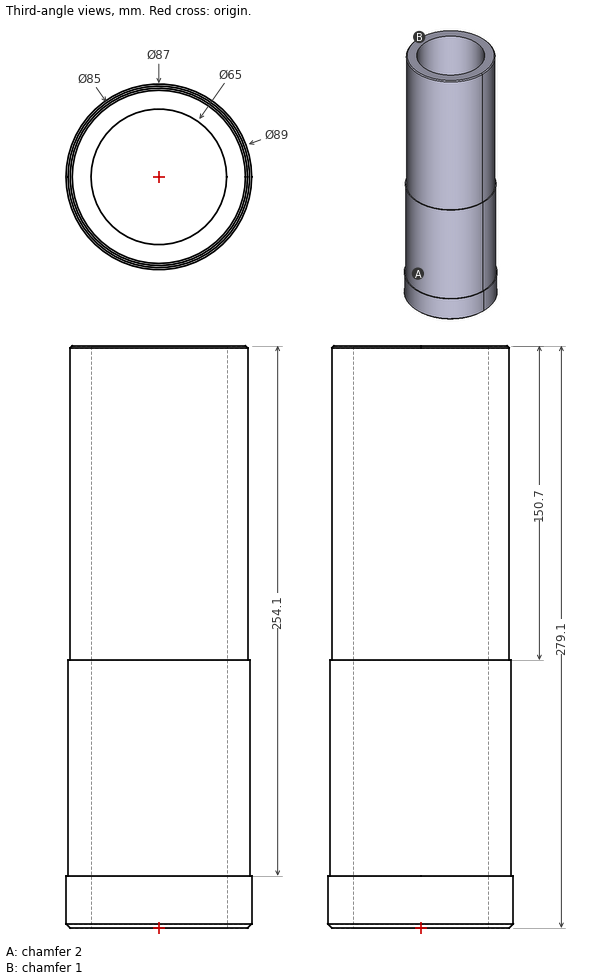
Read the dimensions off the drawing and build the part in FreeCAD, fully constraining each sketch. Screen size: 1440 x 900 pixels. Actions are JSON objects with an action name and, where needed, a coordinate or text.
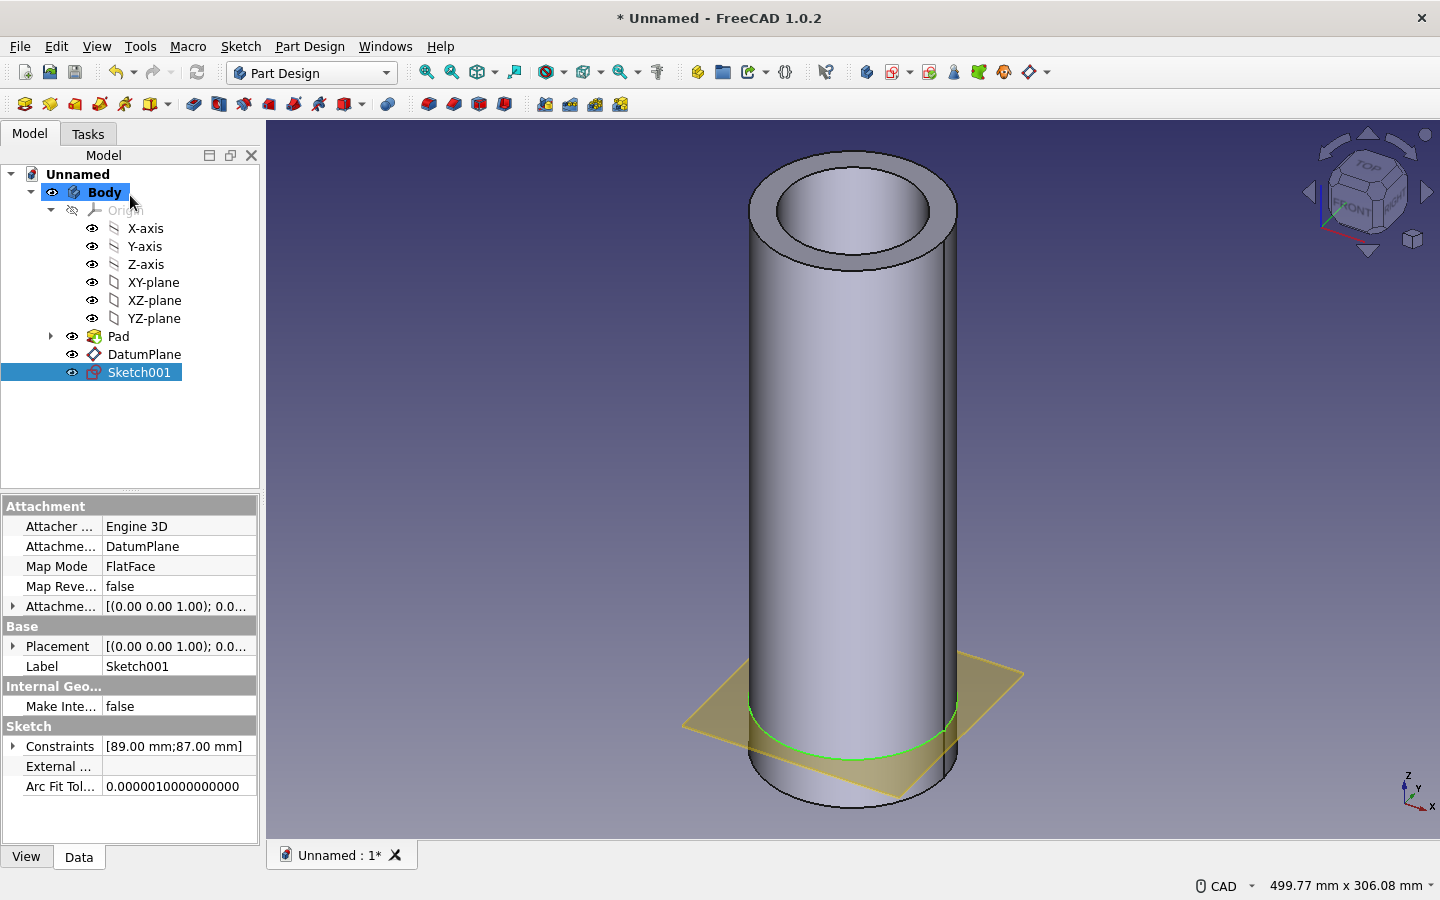
{"action": "left_click", "coordinate": [194, 104]}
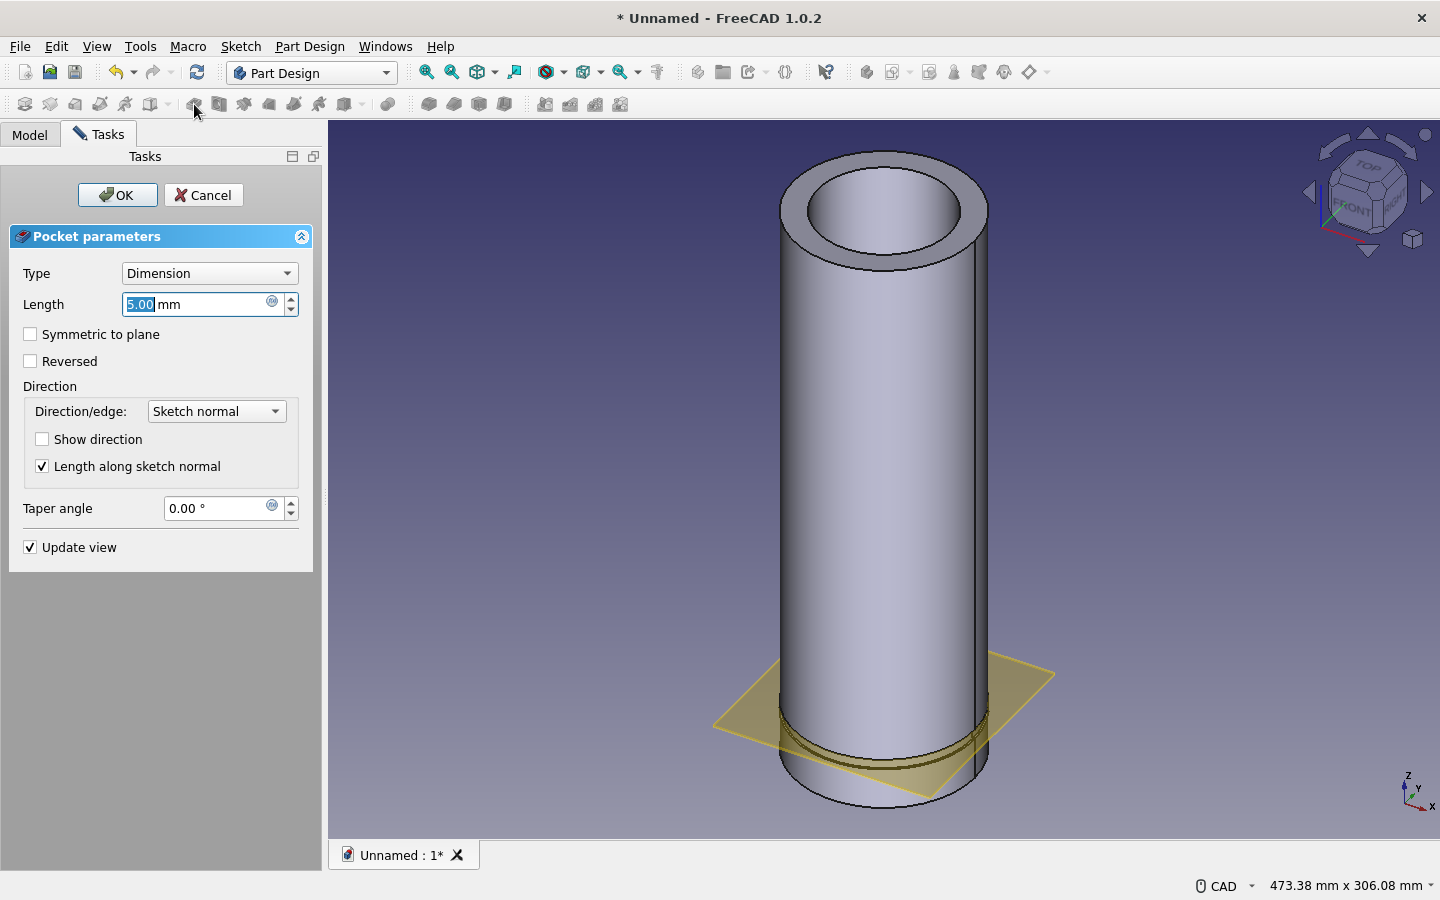
{"action": "type", "text": "254.1"}
{"action": "key", "text": "Tab"}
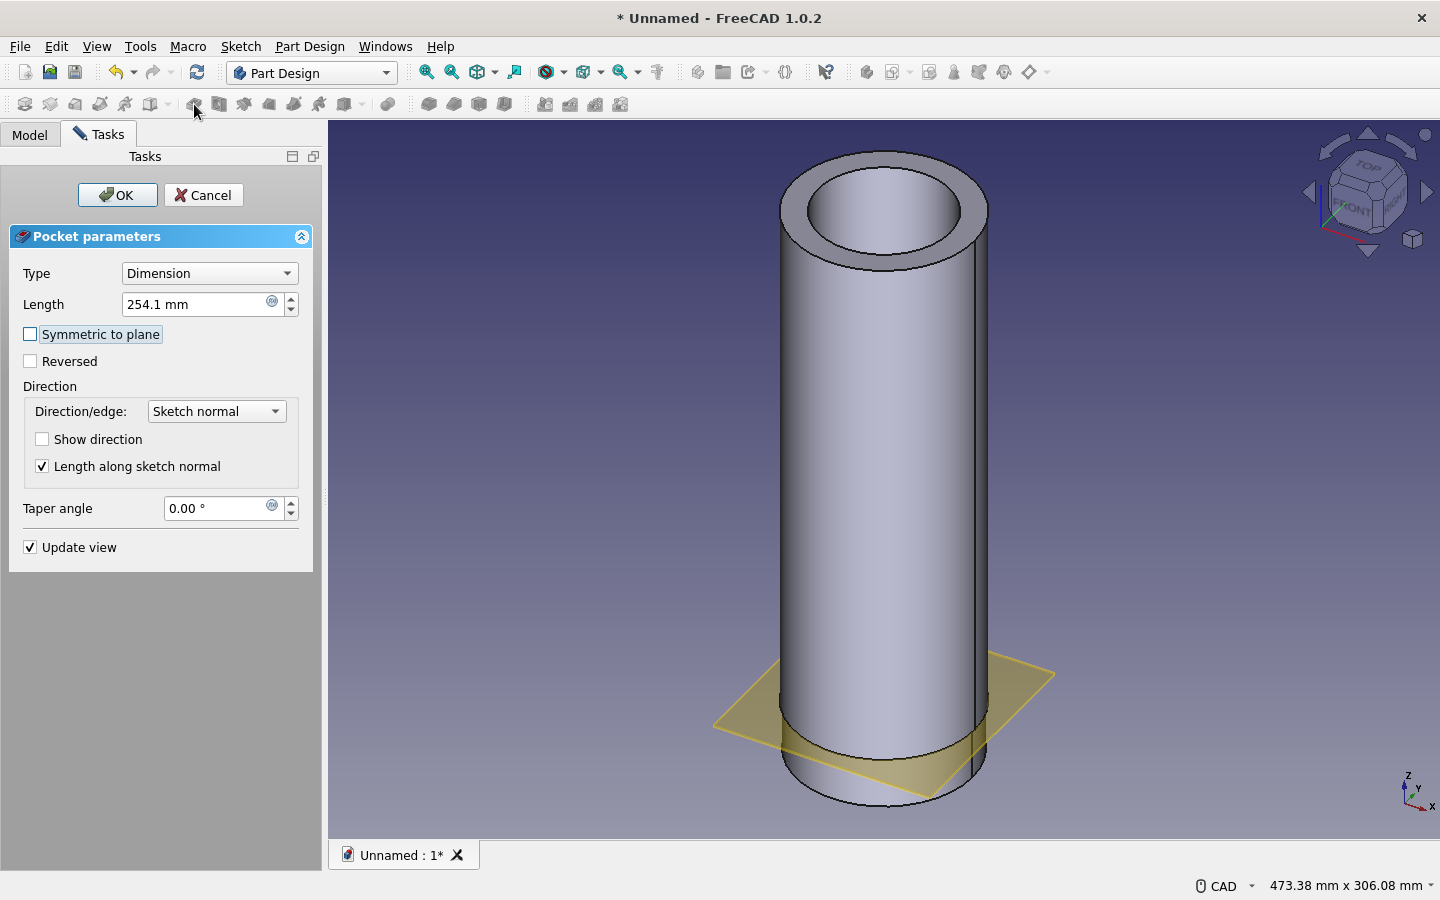
{"action": "left_click", "coordinate": [31, 361]}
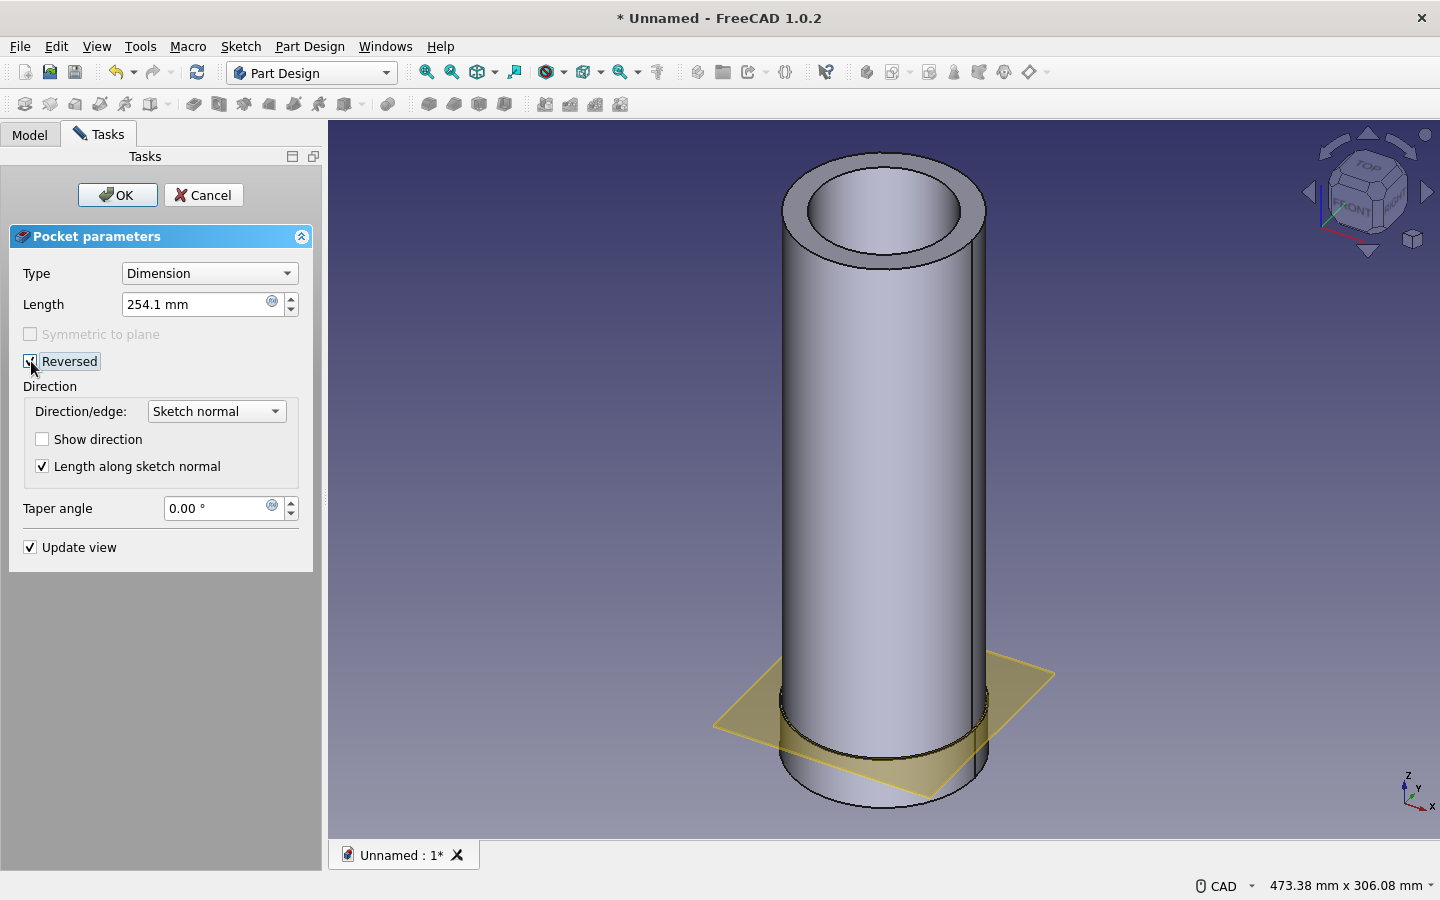
{"action": "left_click", "coordinate": [118, 195]}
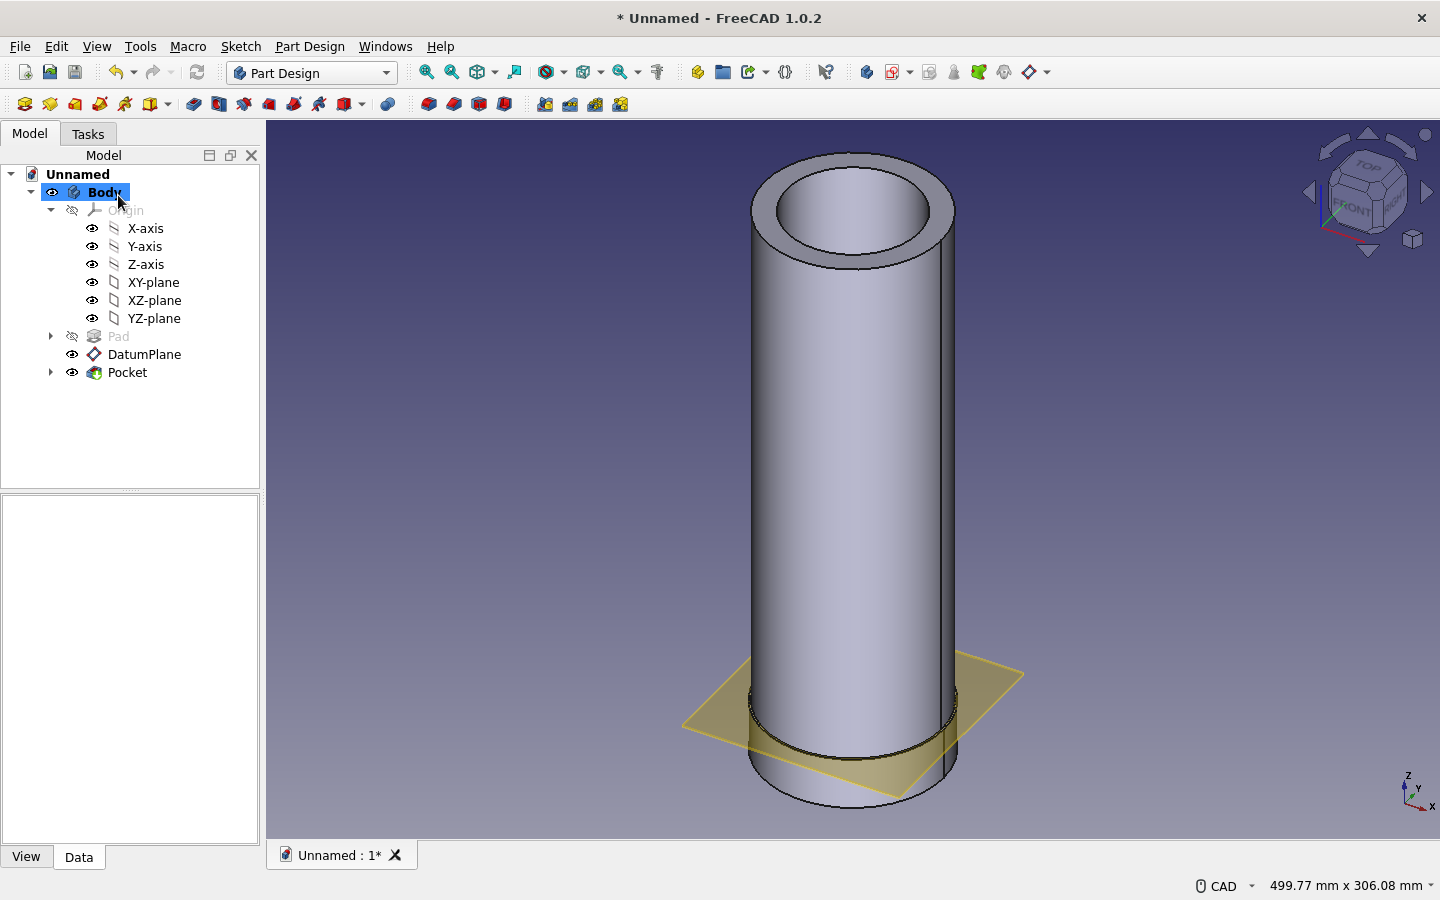
{"action": "left_click", "coordinate": [117, 354]}
{"action": "key", "text": "space"}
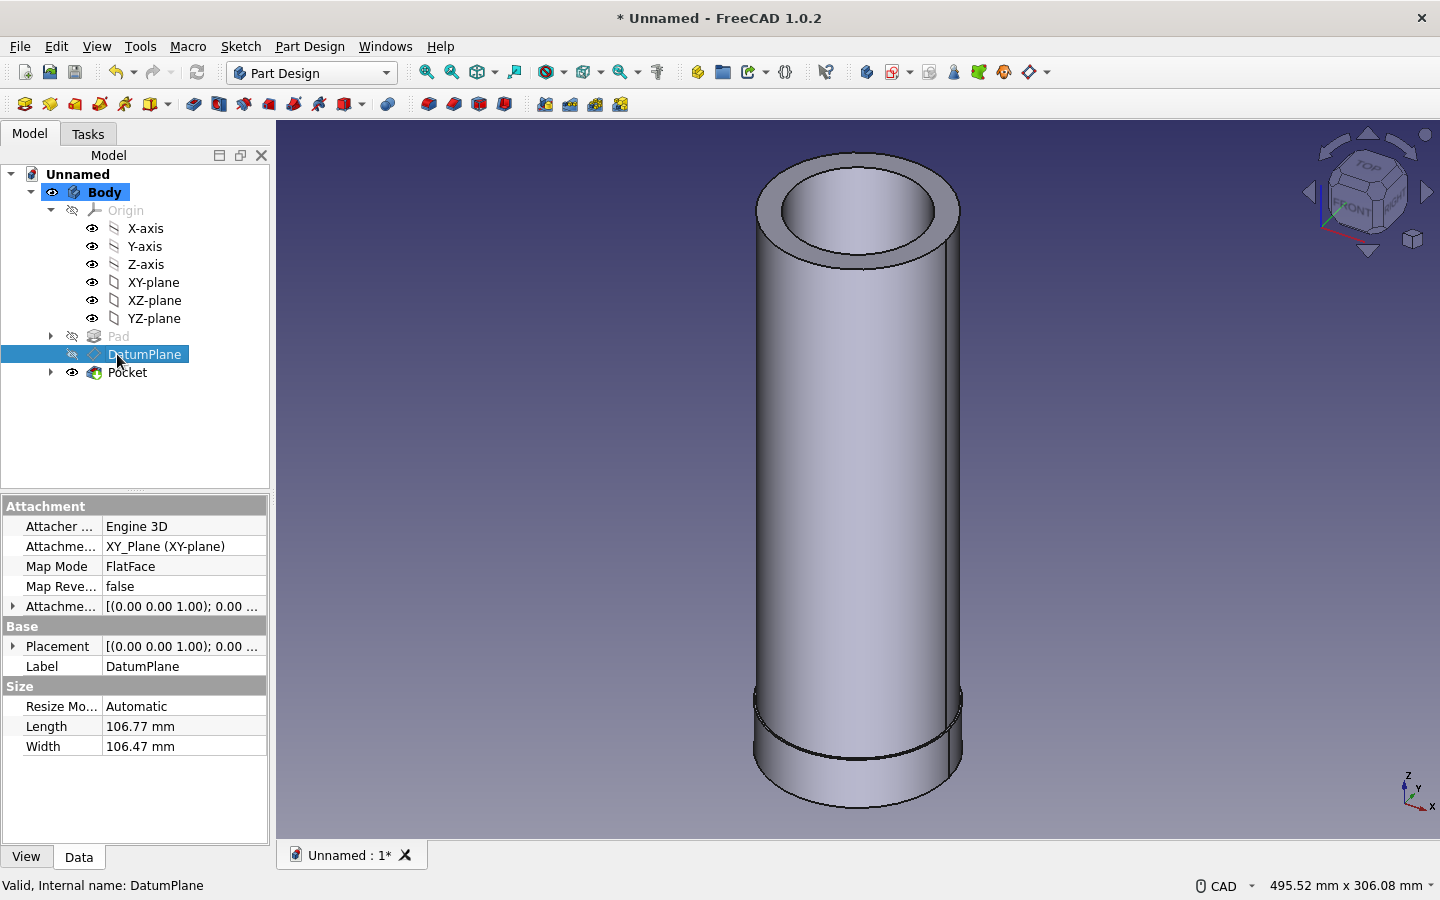
{"action": "left_click", "coordinate": [137, 282]}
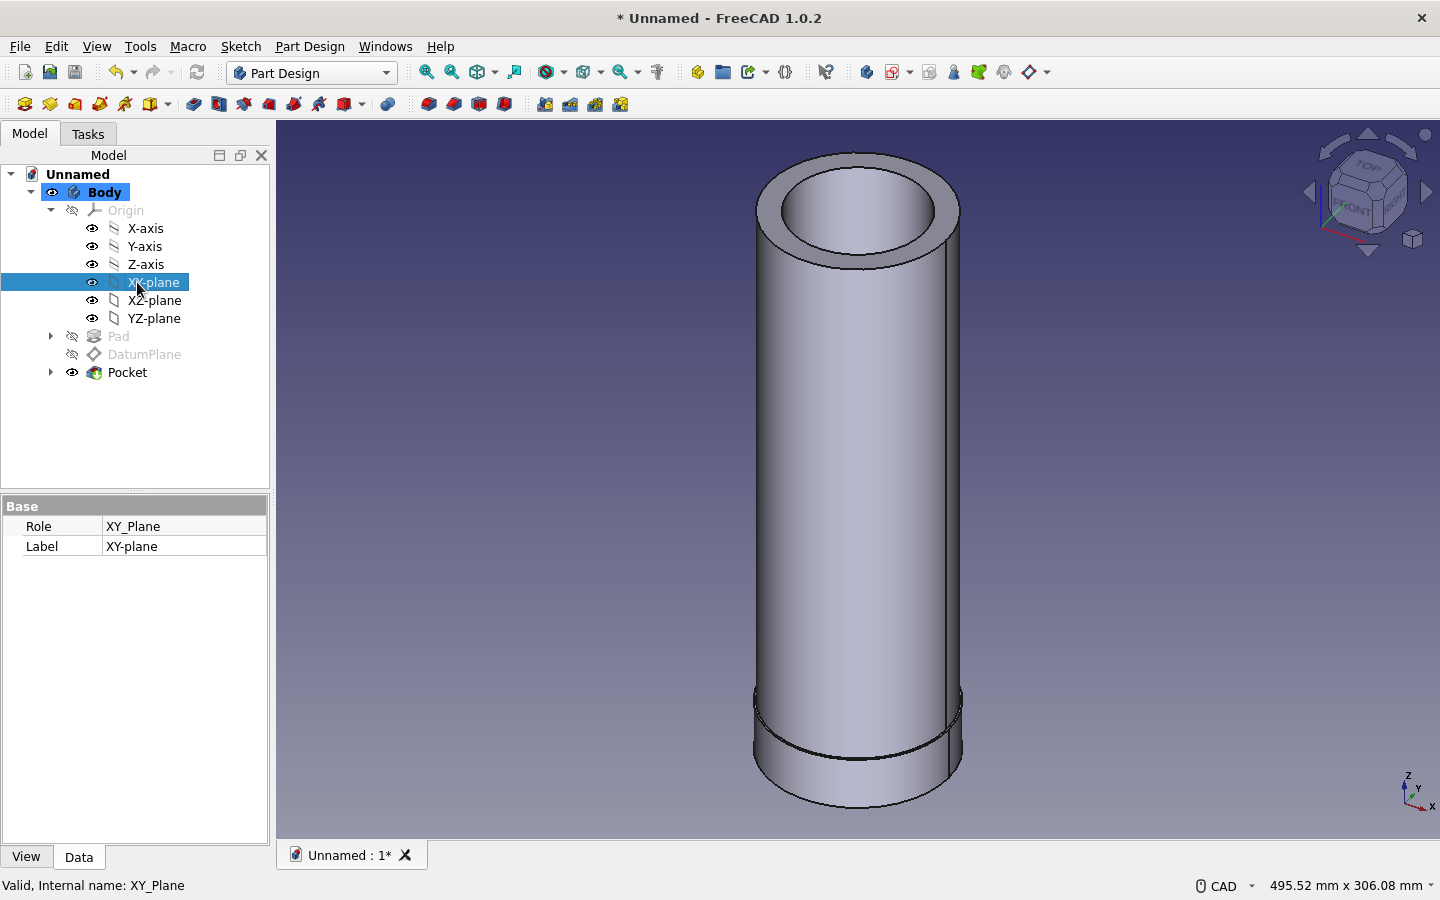
{"action": "left_click", "coordinate": [1028, 72]}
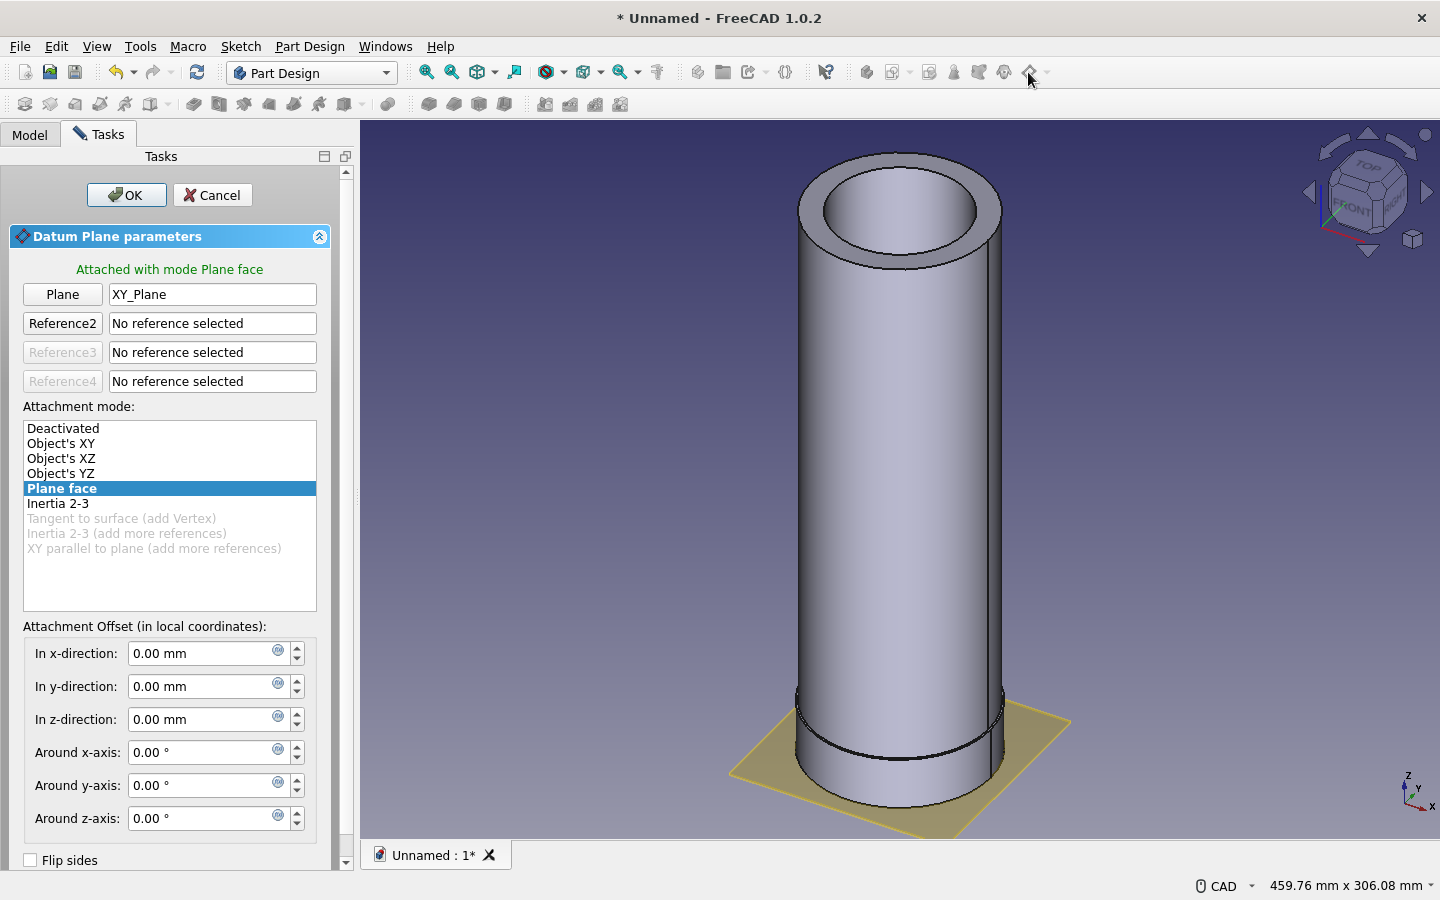
{"action": "triple_click", "coordinate": [210, 720]}